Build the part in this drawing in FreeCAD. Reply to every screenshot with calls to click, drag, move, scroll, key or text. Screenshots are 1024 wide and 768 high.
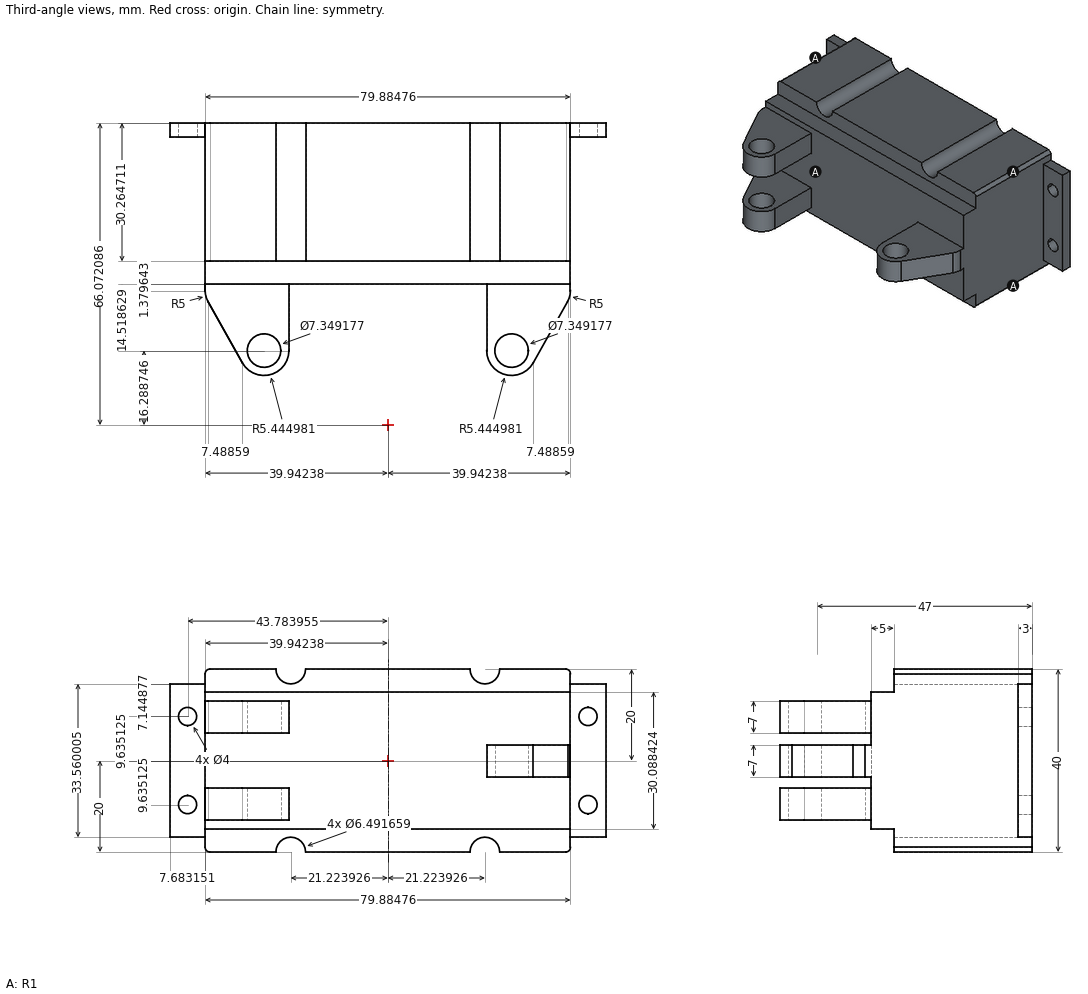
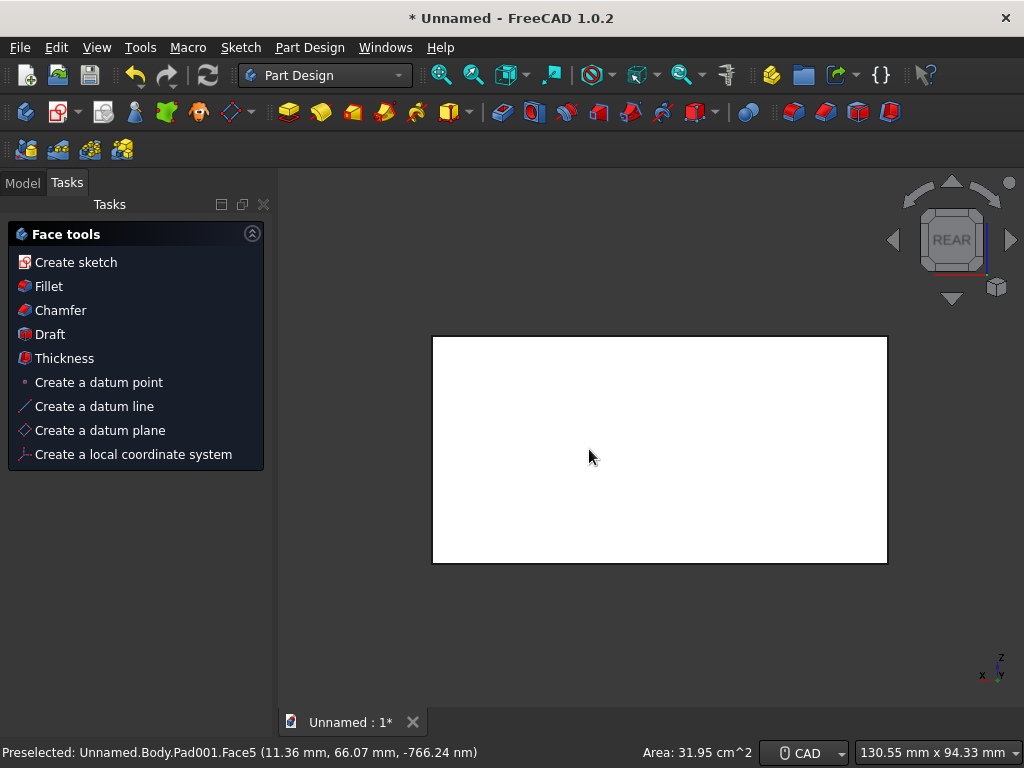
click(58, 112)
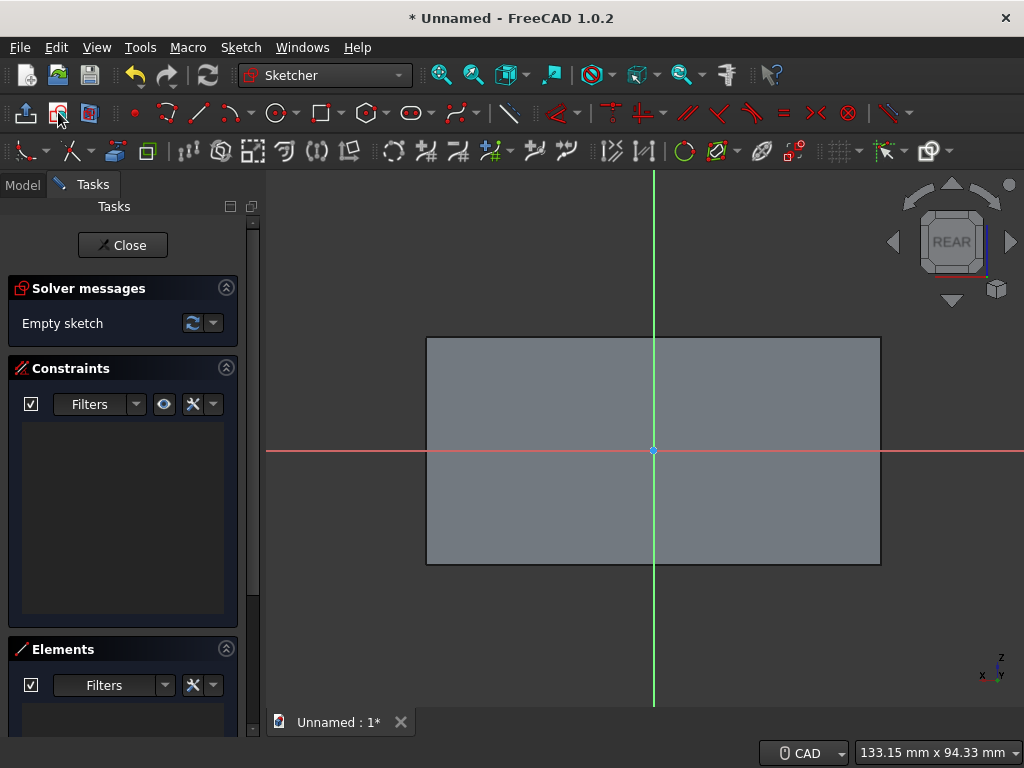
key(g)
key(c)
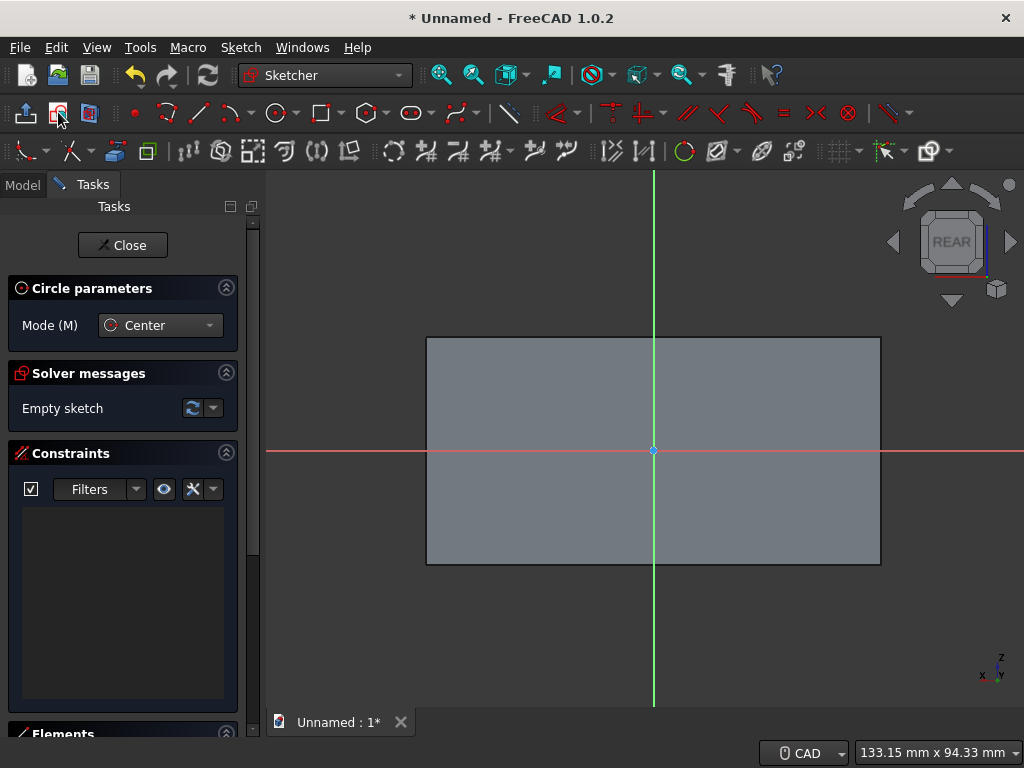
scroll(775, 565, up, 2)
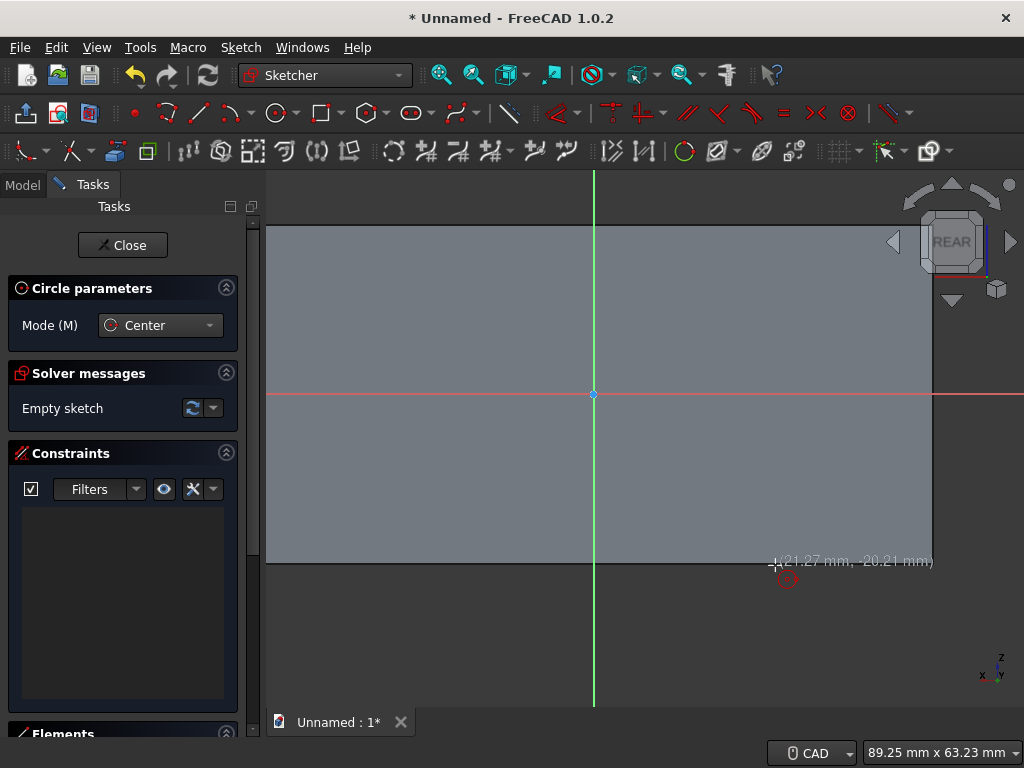
click(774, 564)
click(794, 545)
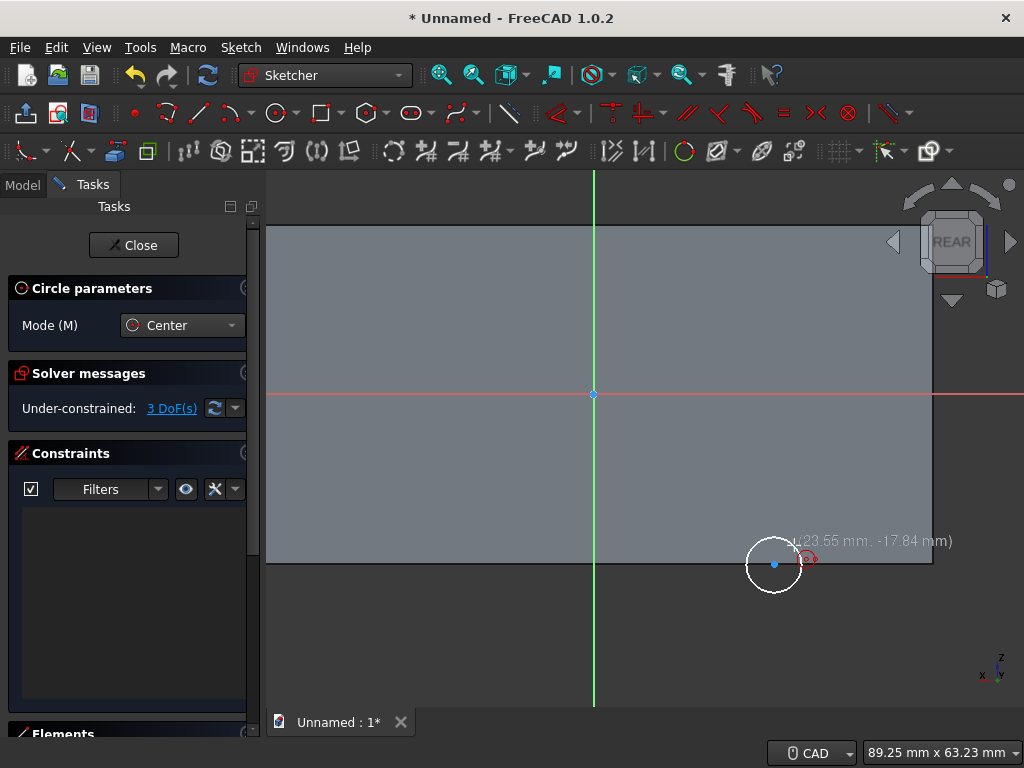
click(414, 564)
click(433, 545)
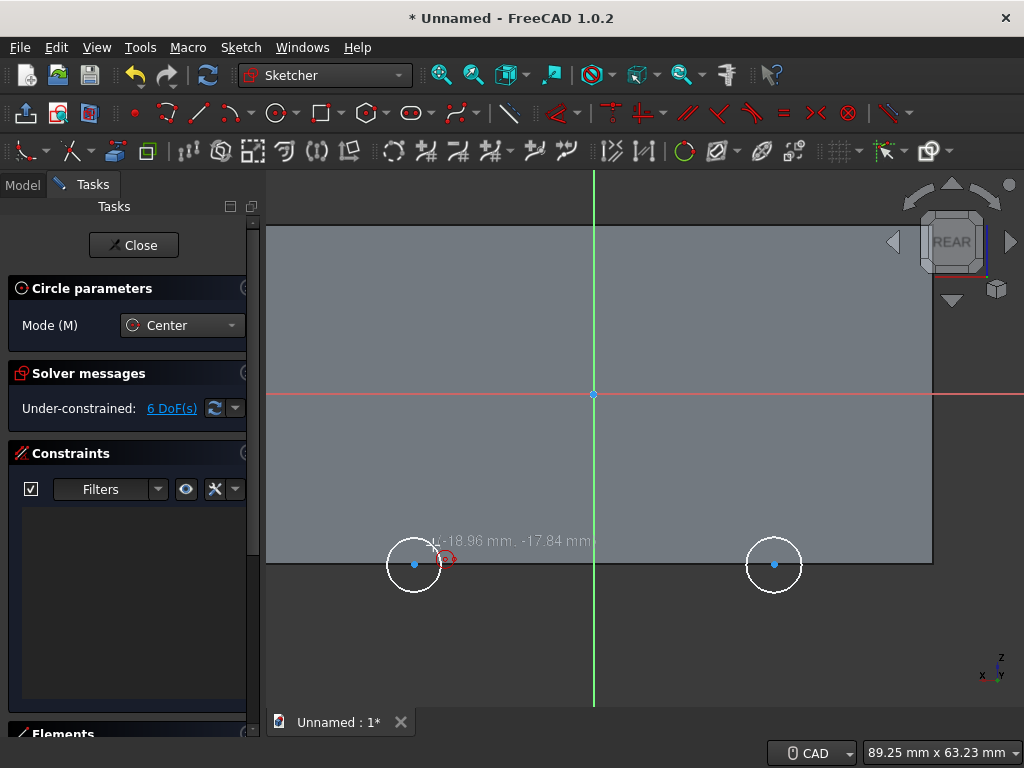
click(414, 225)
click(433, 205)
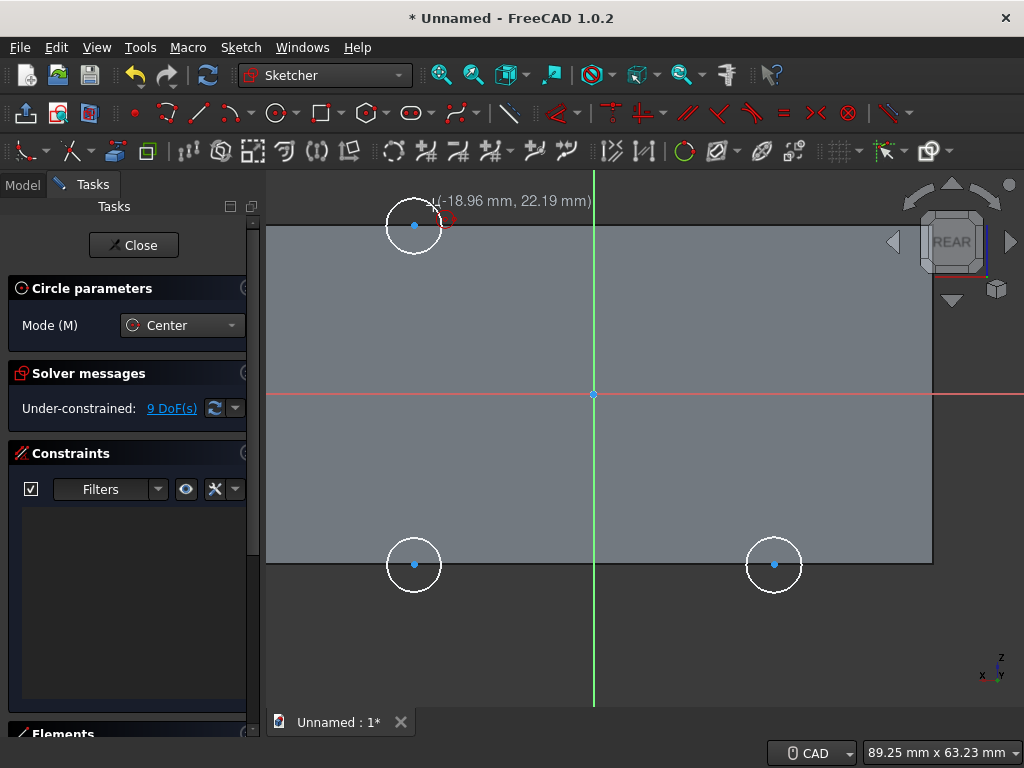
click(774, 225)
click(794, 205)
key(Escape)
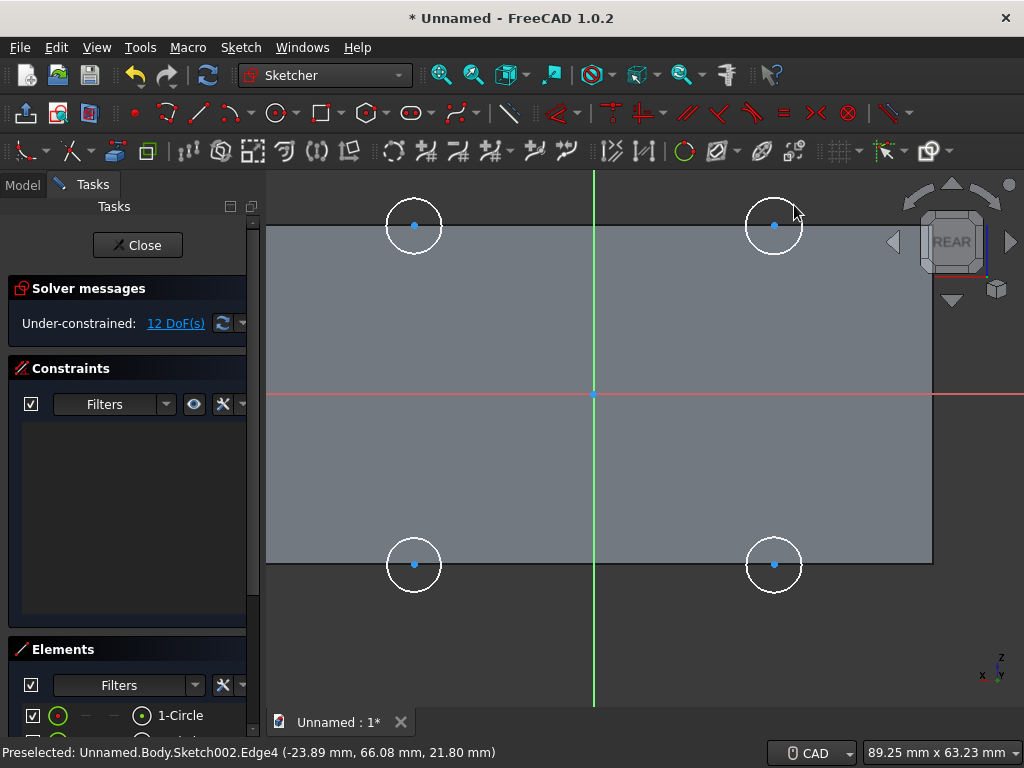
click(793, 545)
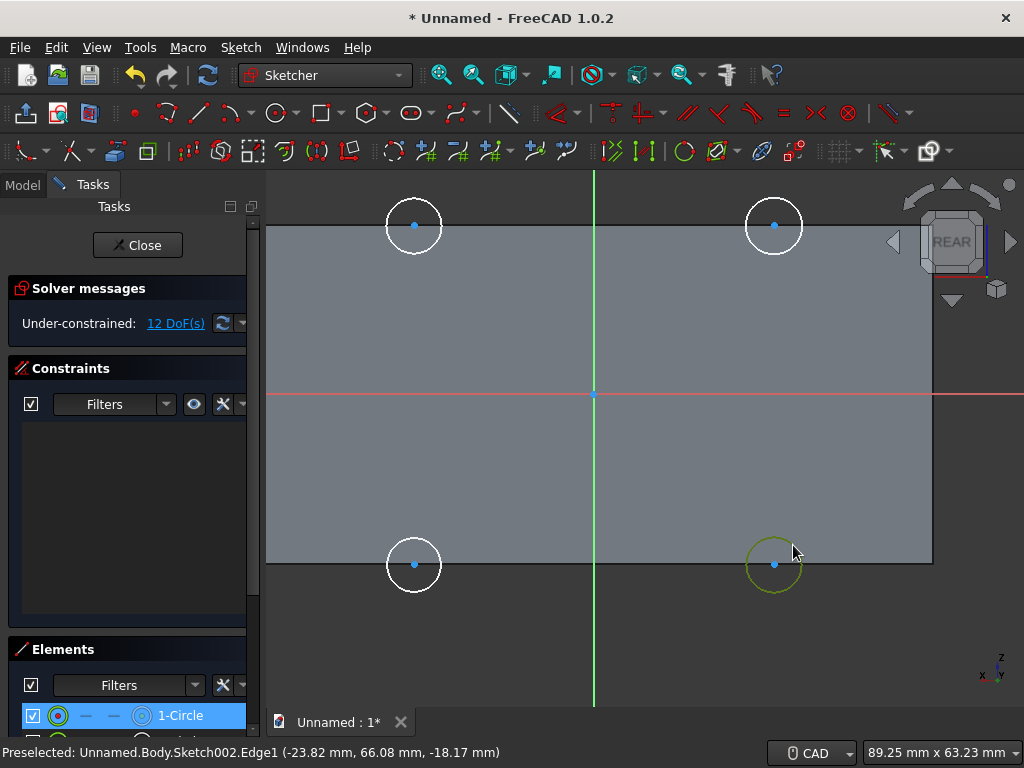
click(433, 546)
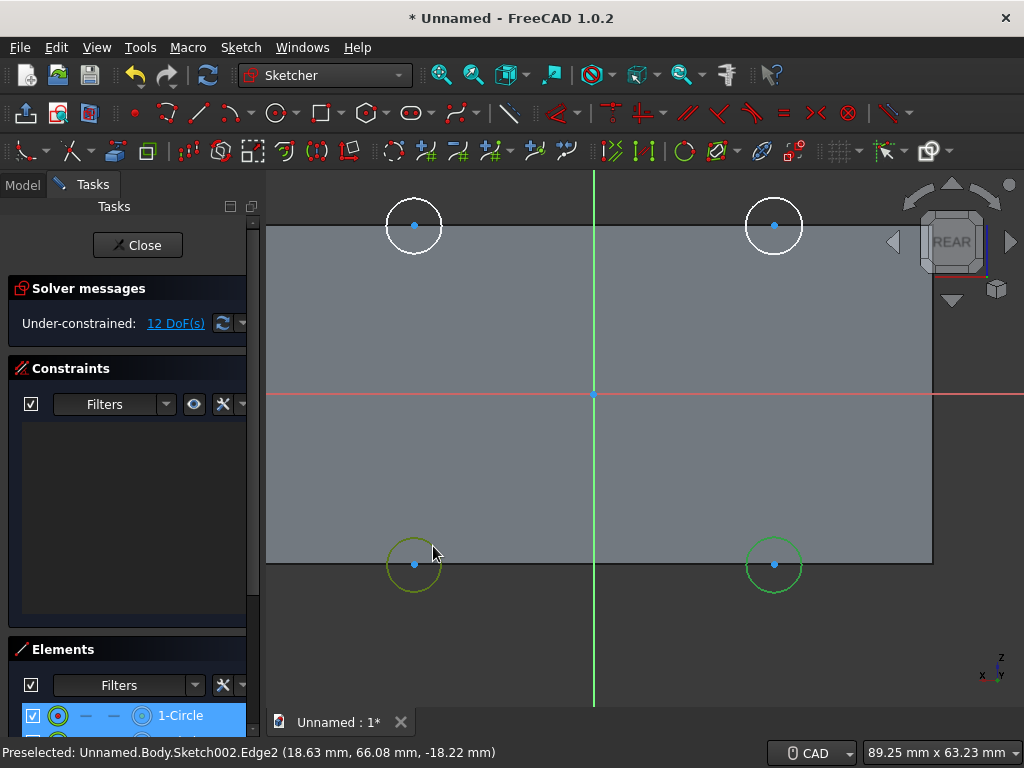
click(433, 206)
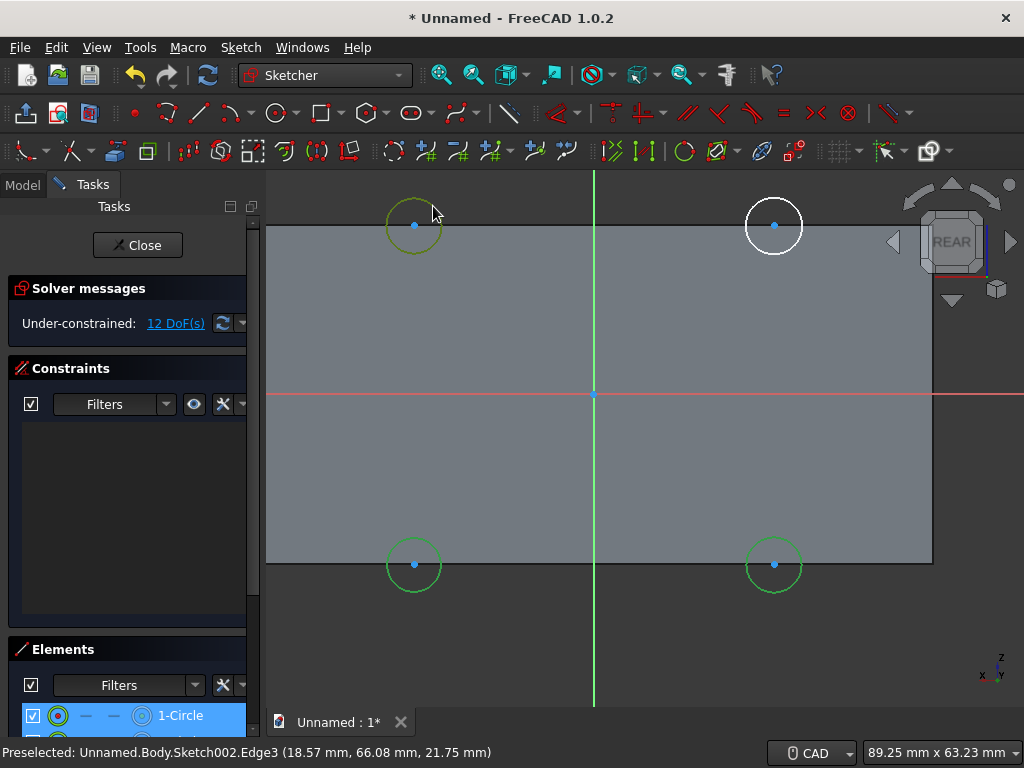
click(794, 206)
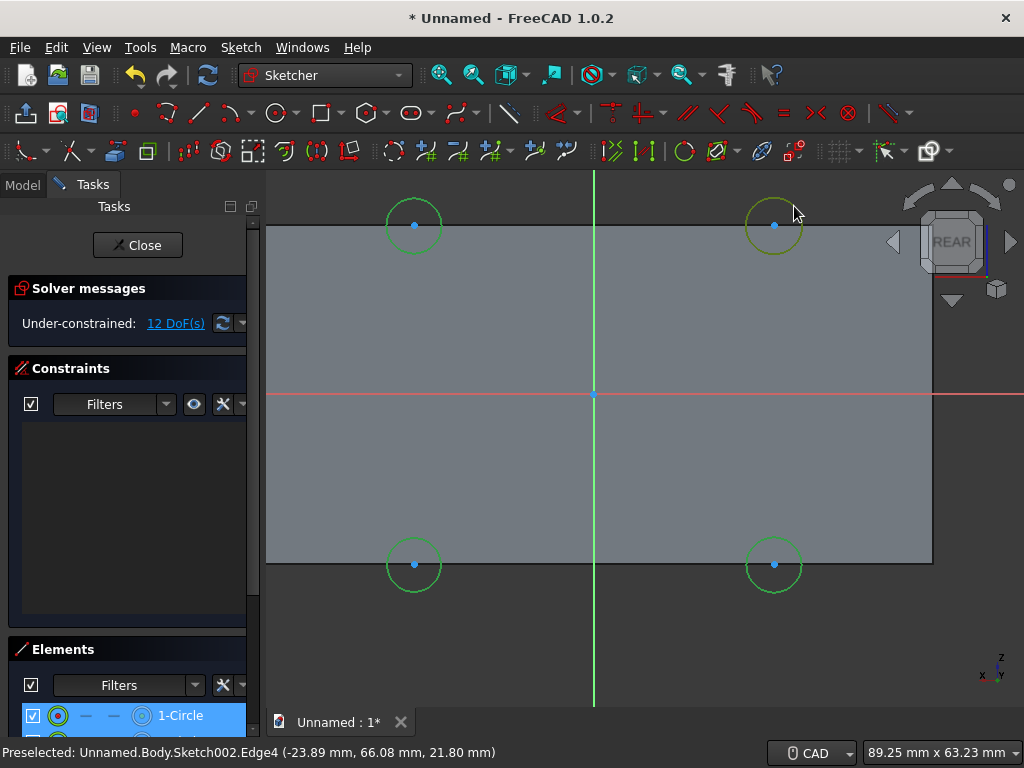
click(784, 114)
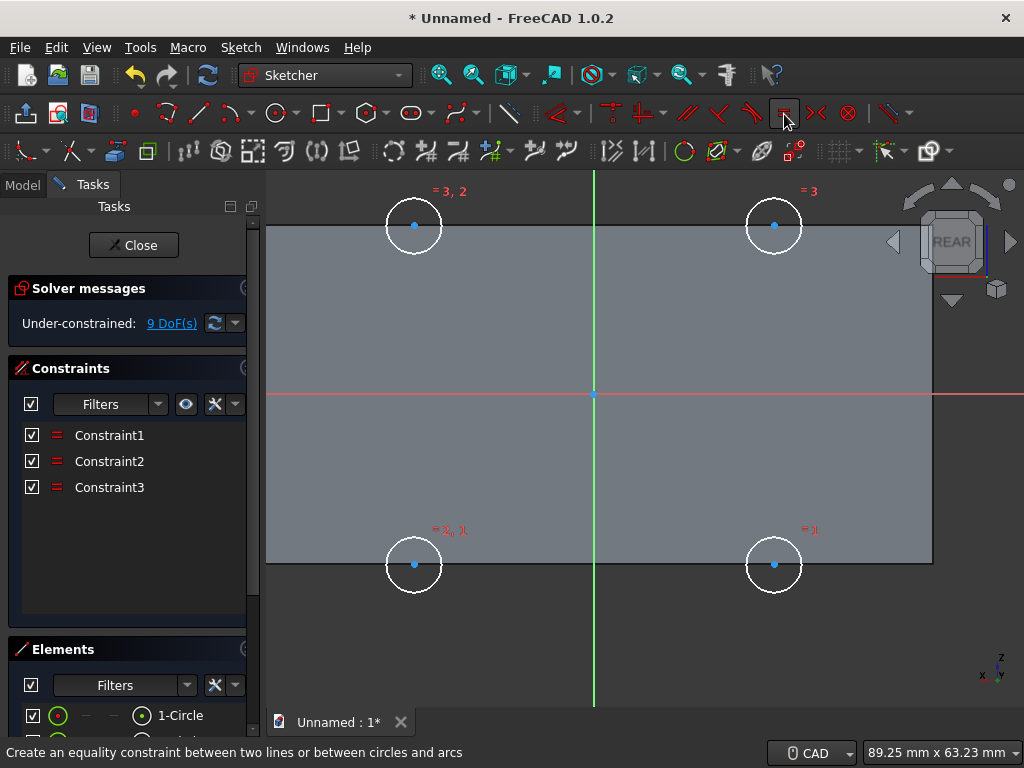
click(774, 565)